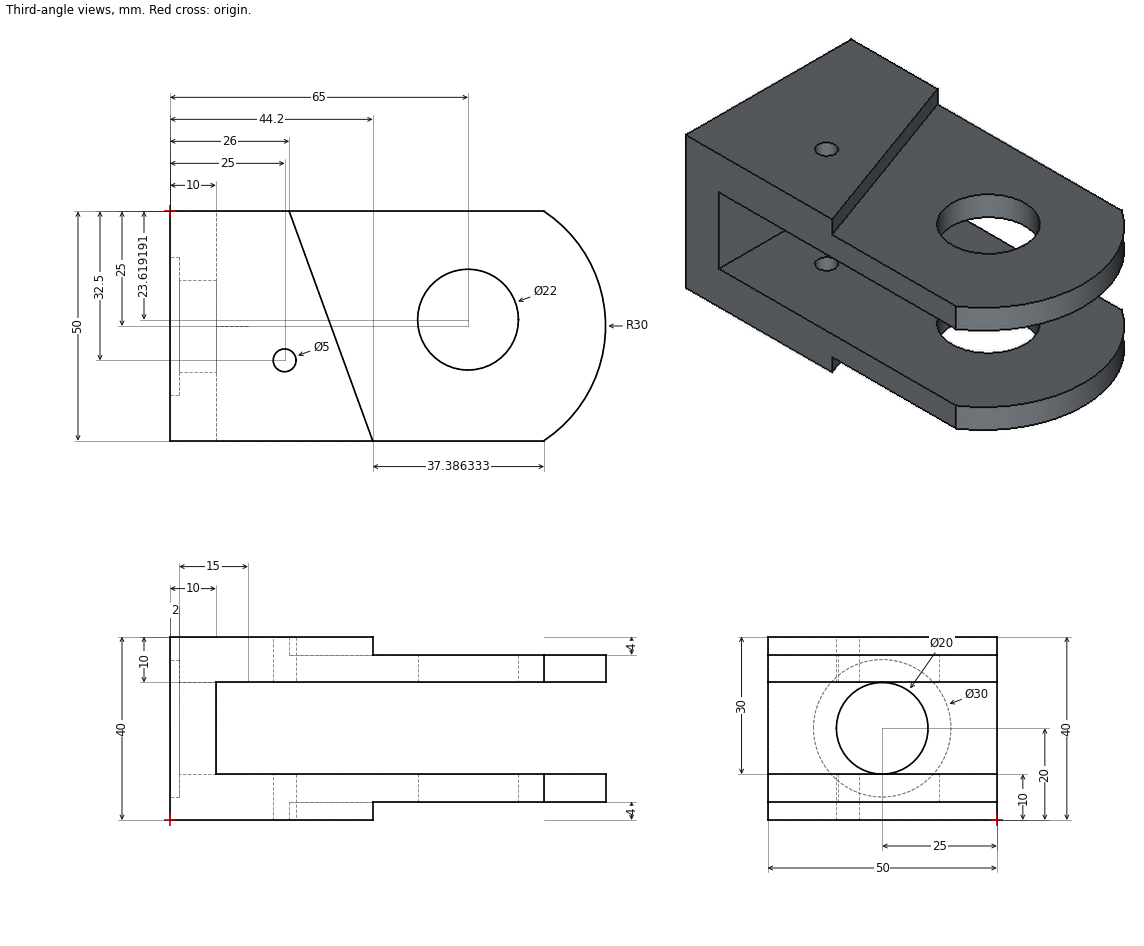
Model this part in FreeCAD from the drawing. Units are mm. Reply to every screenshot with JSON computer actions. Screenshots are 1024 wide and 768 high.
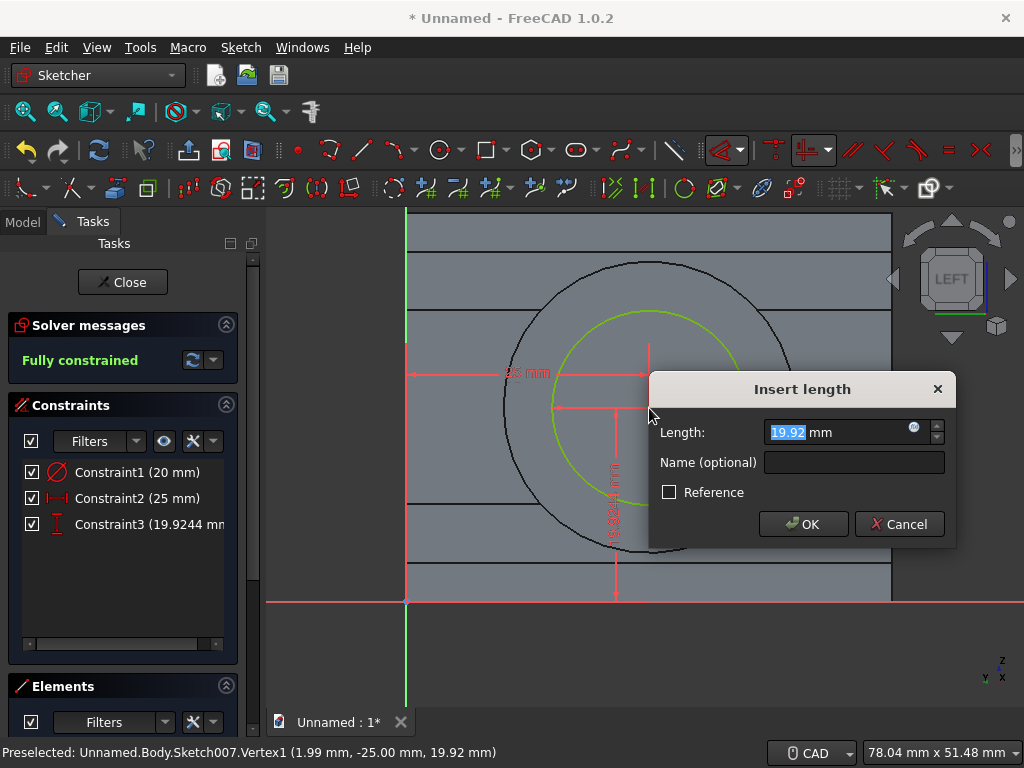
{"action": "type", "text": "20"}
{"action": "key", "text": "Return"}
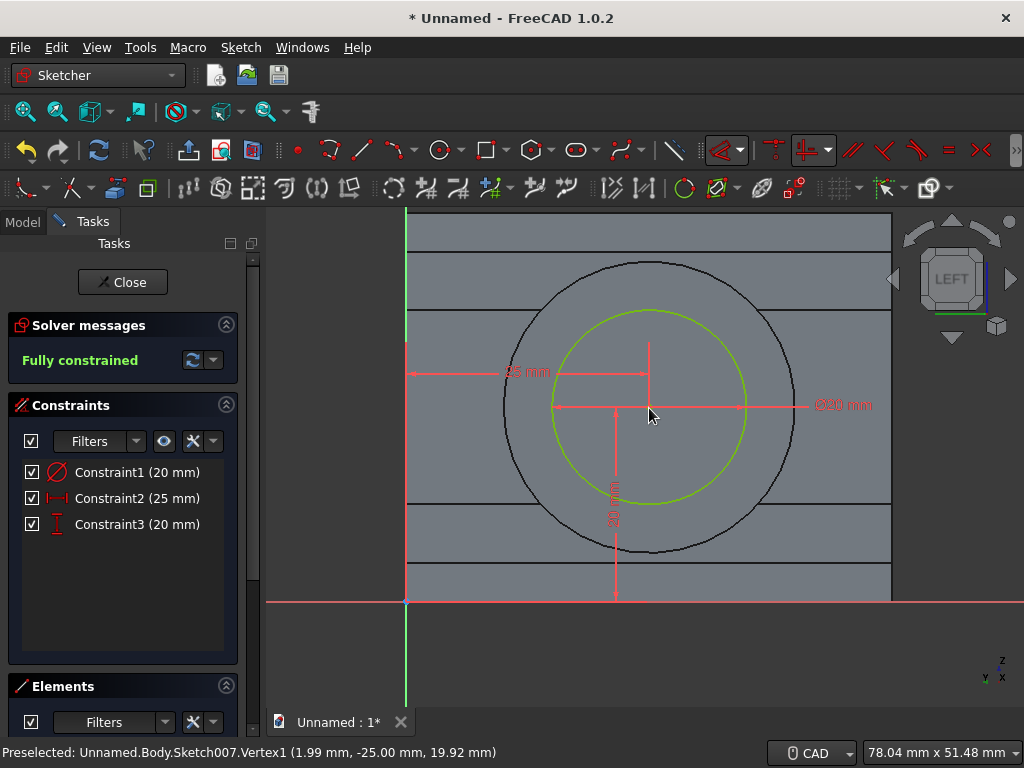
{"action": "left_click", "coordinate": [123, 282]}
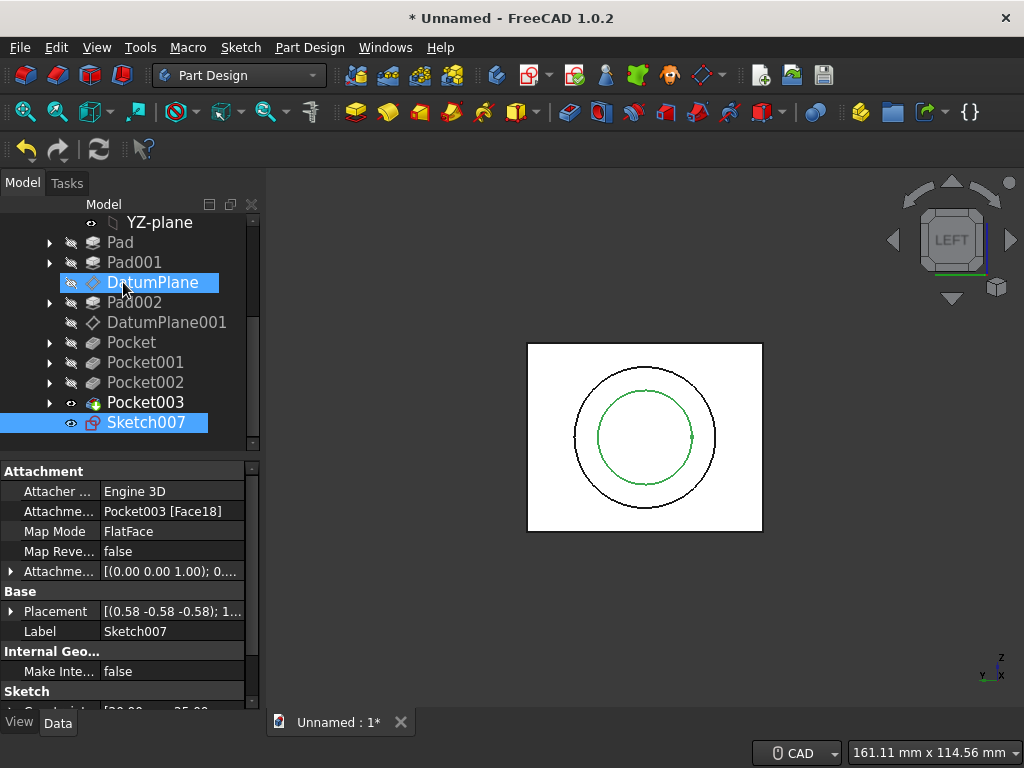
{"action": "left_click", "coordinate": [570, 112]}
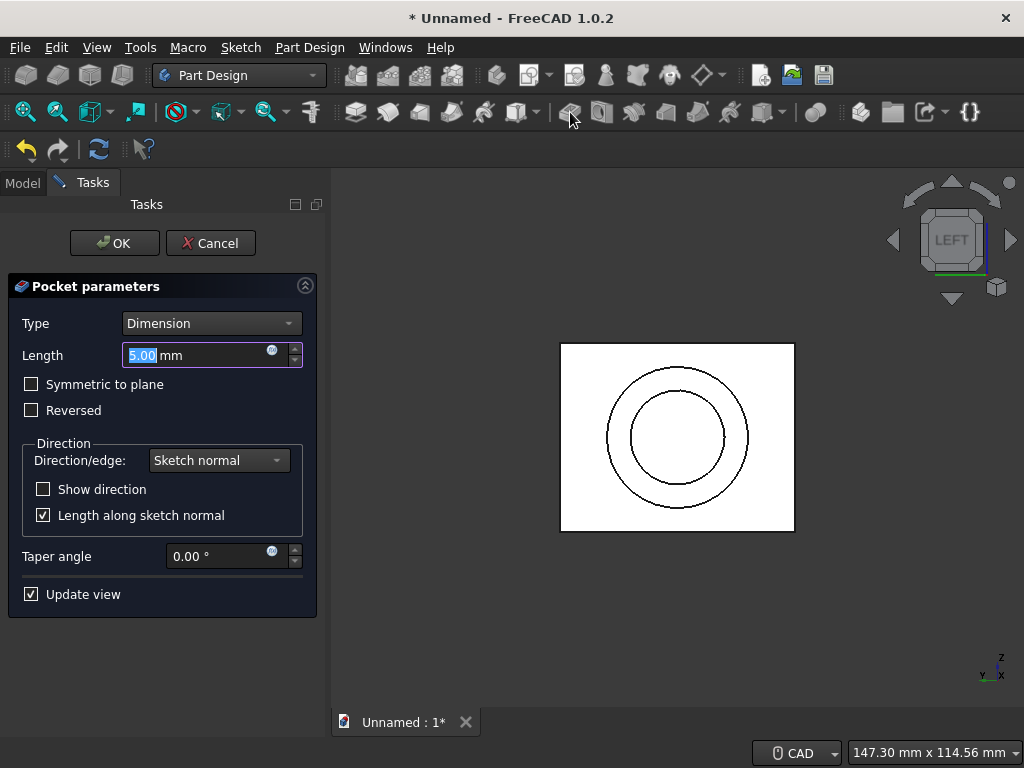
{"action": "type", "text": "15"}
{"action": "key", "text": "Tab"}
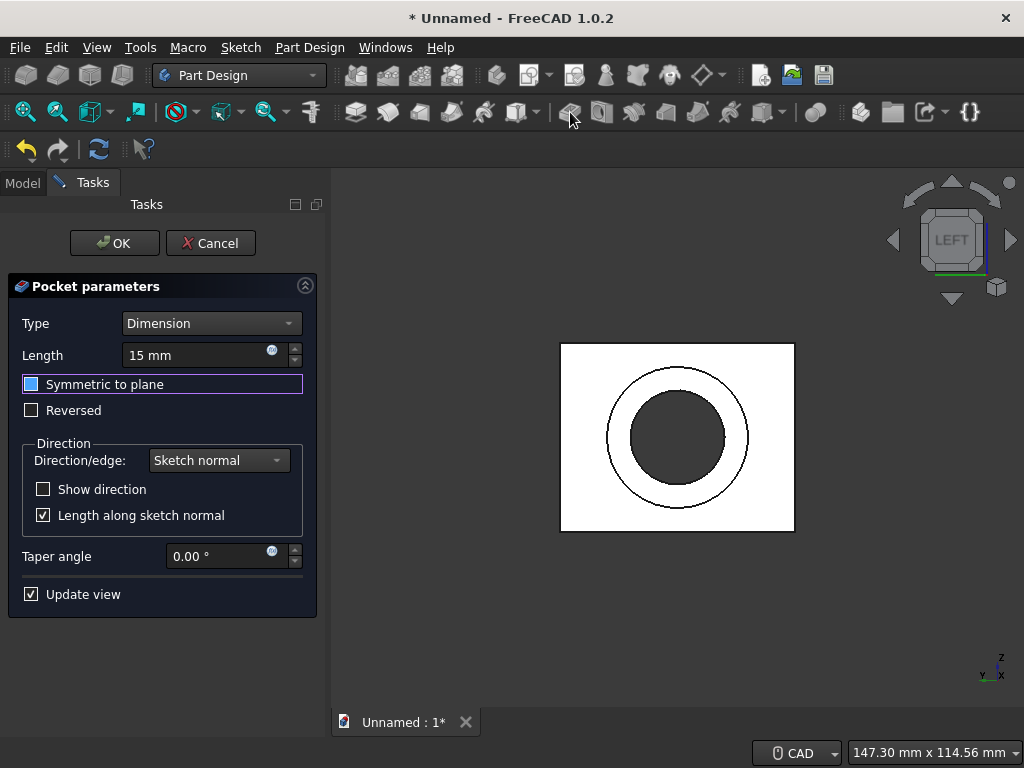
{"action": "left_click", "coordinate": [115, 243]}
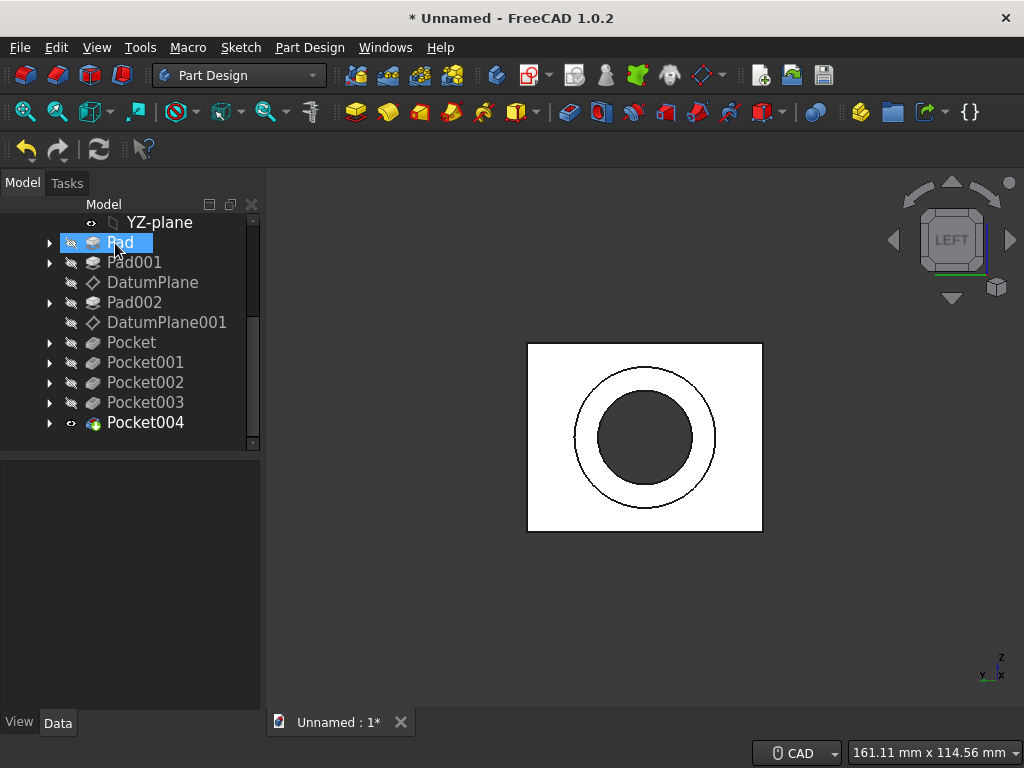
{"action": "left_click", "coordinate": [26, 112]}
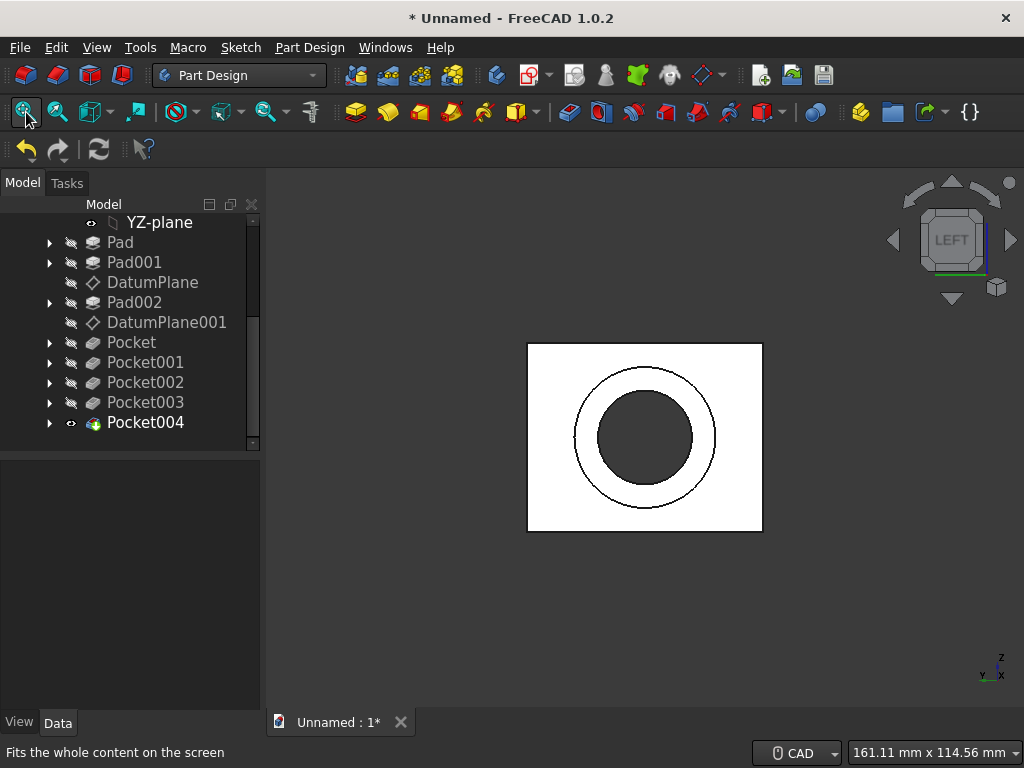
{"action": "key", "text": "0"}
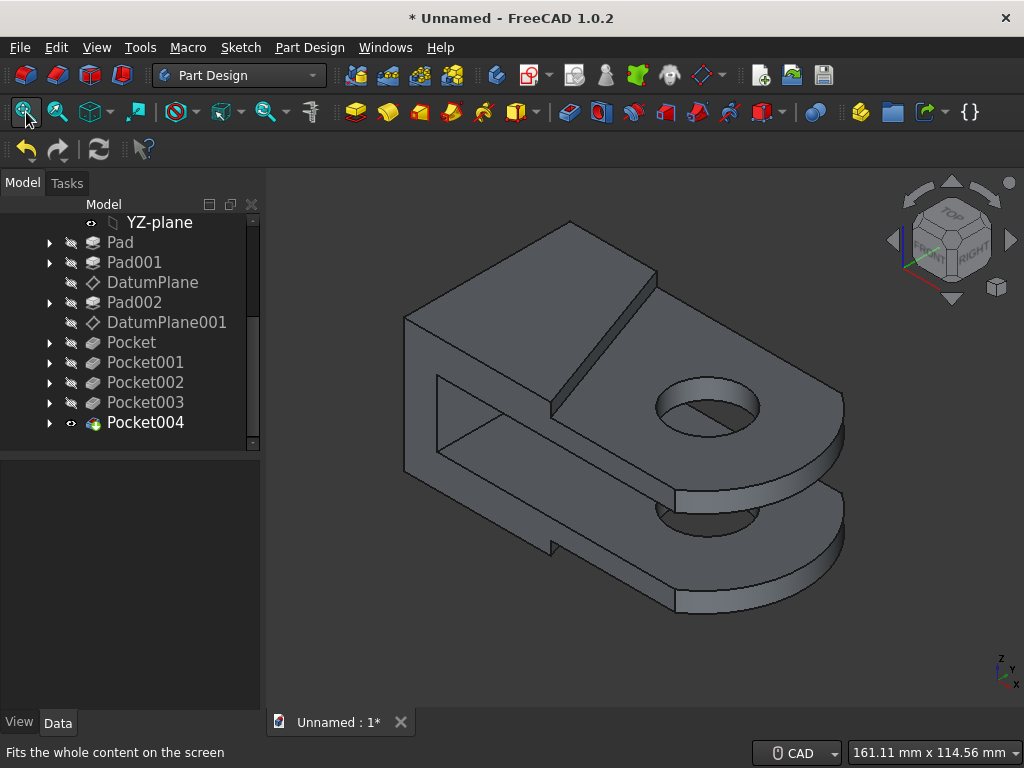
{"action": "left_click", "coordinate": [539, 299]}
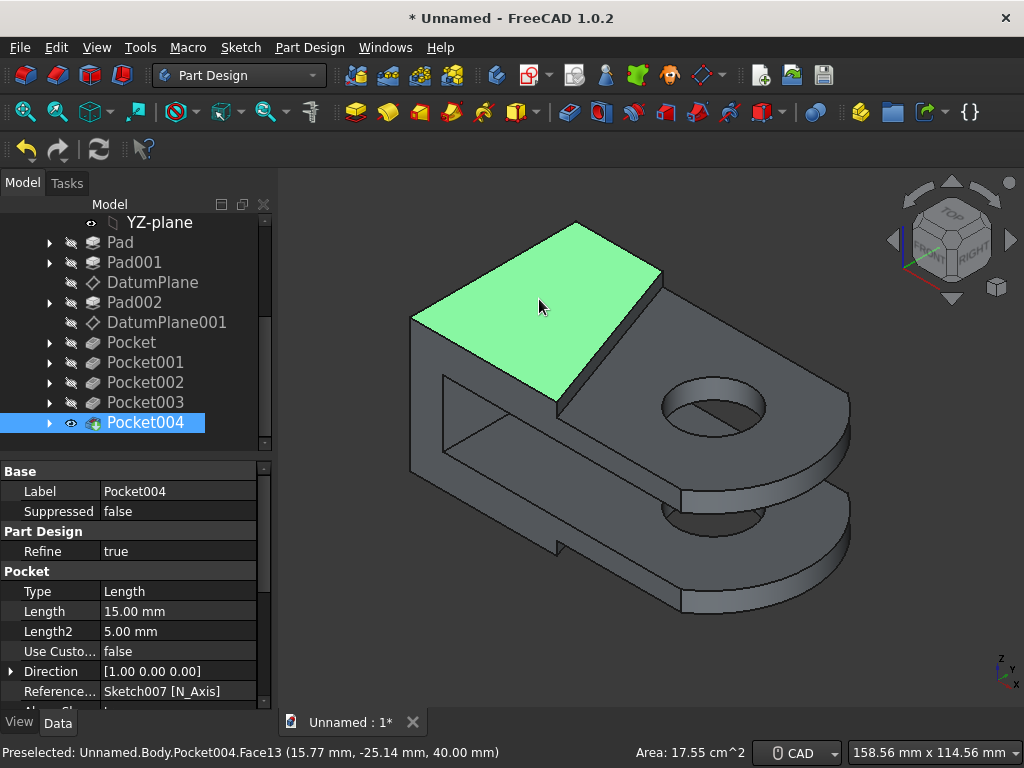
{"action": "left_click", "coordinate": [530, 76]}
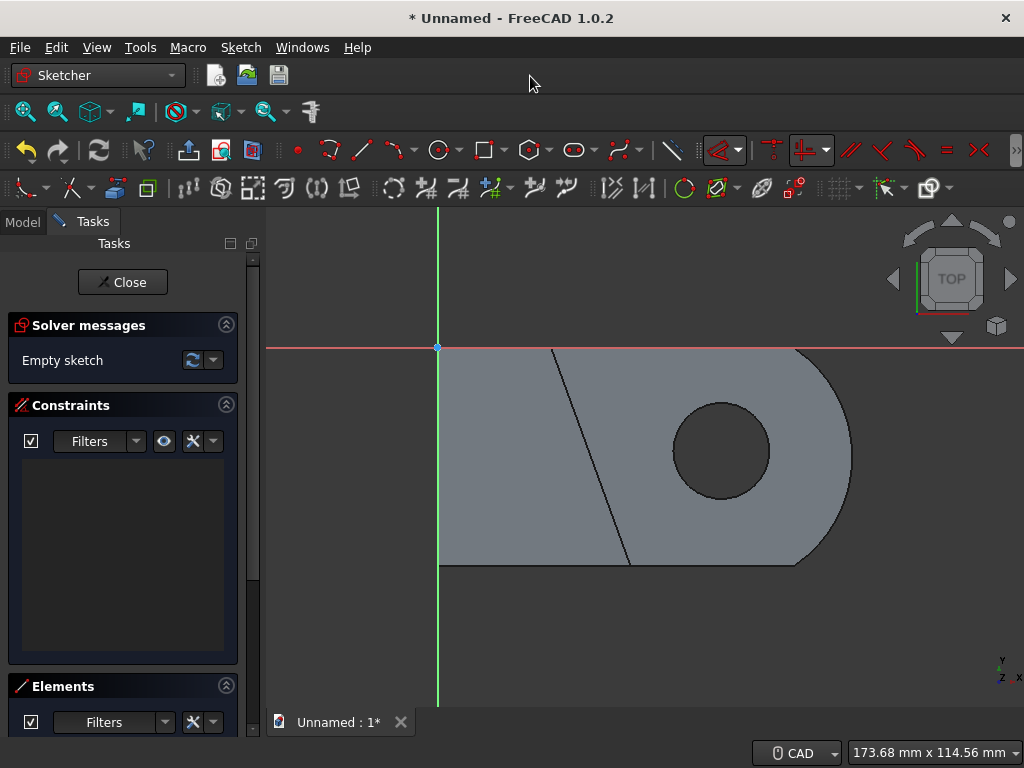
{"action": "scroll", "coordinate": [544, 492], "scroll_direction": "up", "scroll_amount": 13}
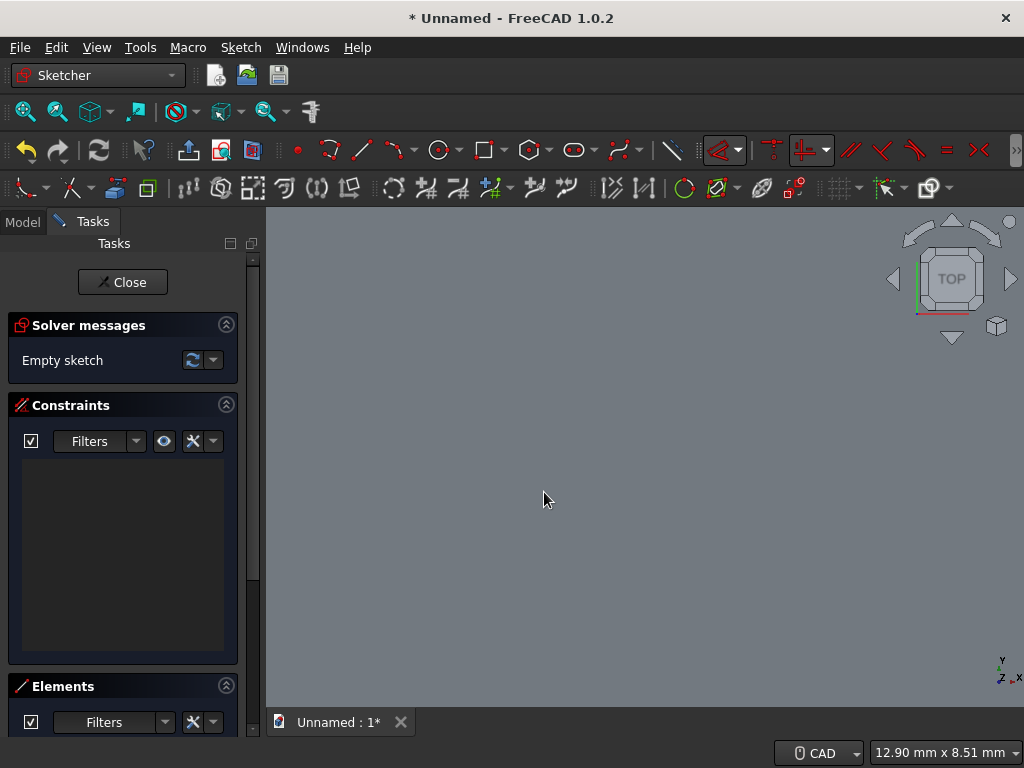
{"action": "left_click", "coordinate": [440, 150]}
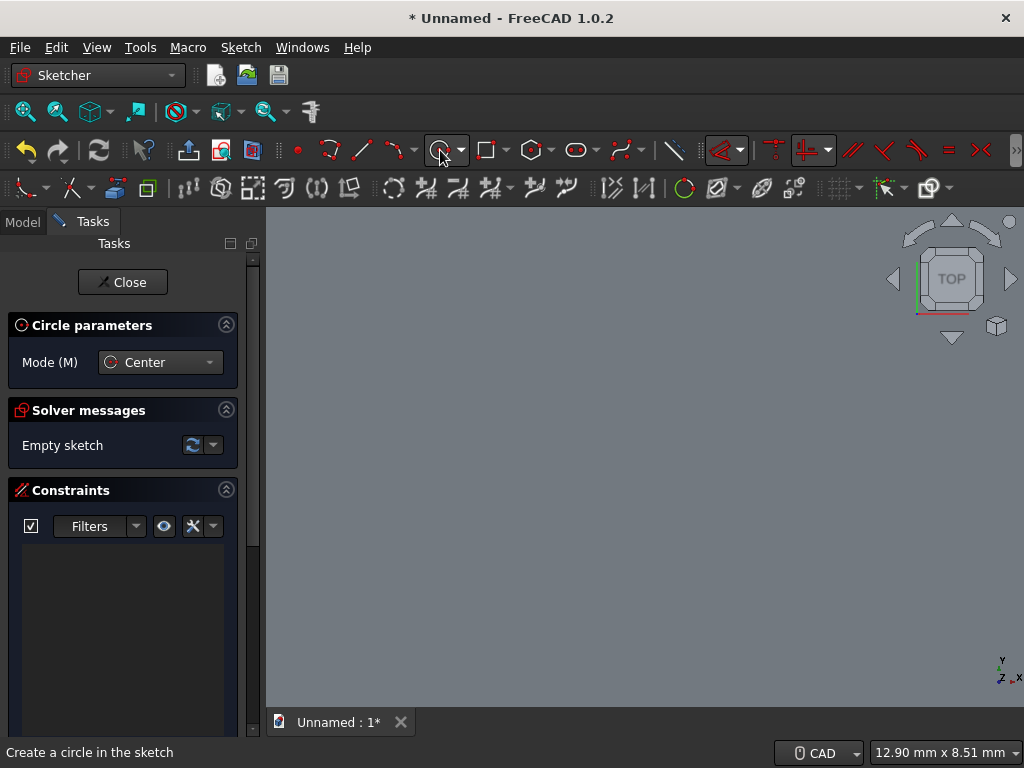
{"action": "left_click", "coordinate": [577, 454]}
{"action": "mouse_move", "coordinate": [681, 350]}